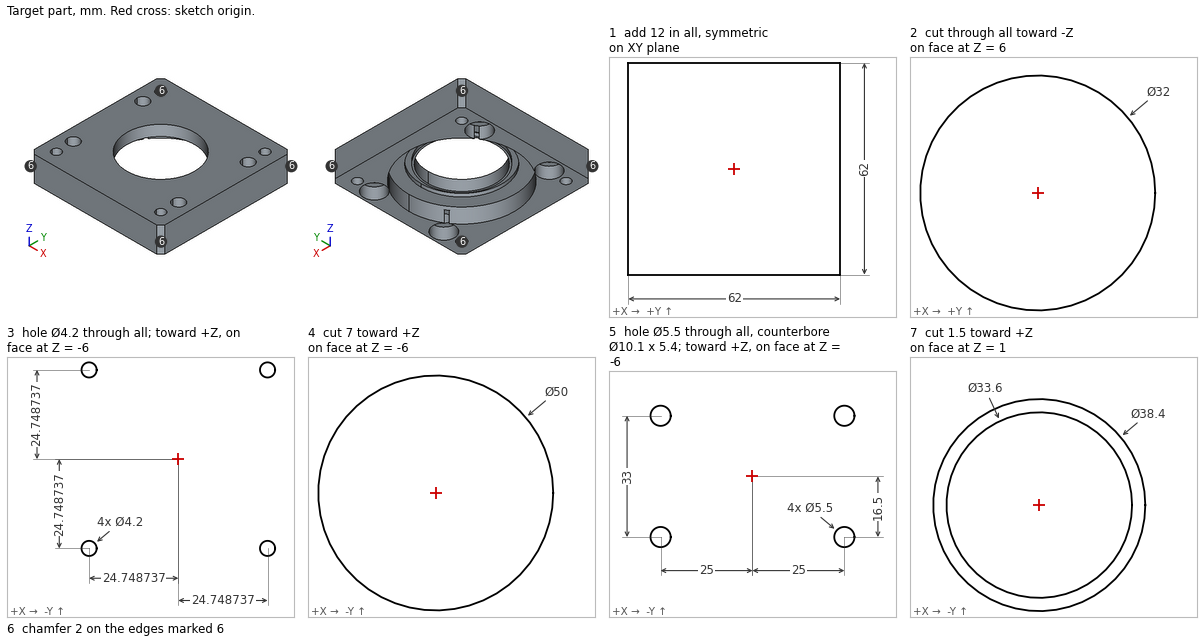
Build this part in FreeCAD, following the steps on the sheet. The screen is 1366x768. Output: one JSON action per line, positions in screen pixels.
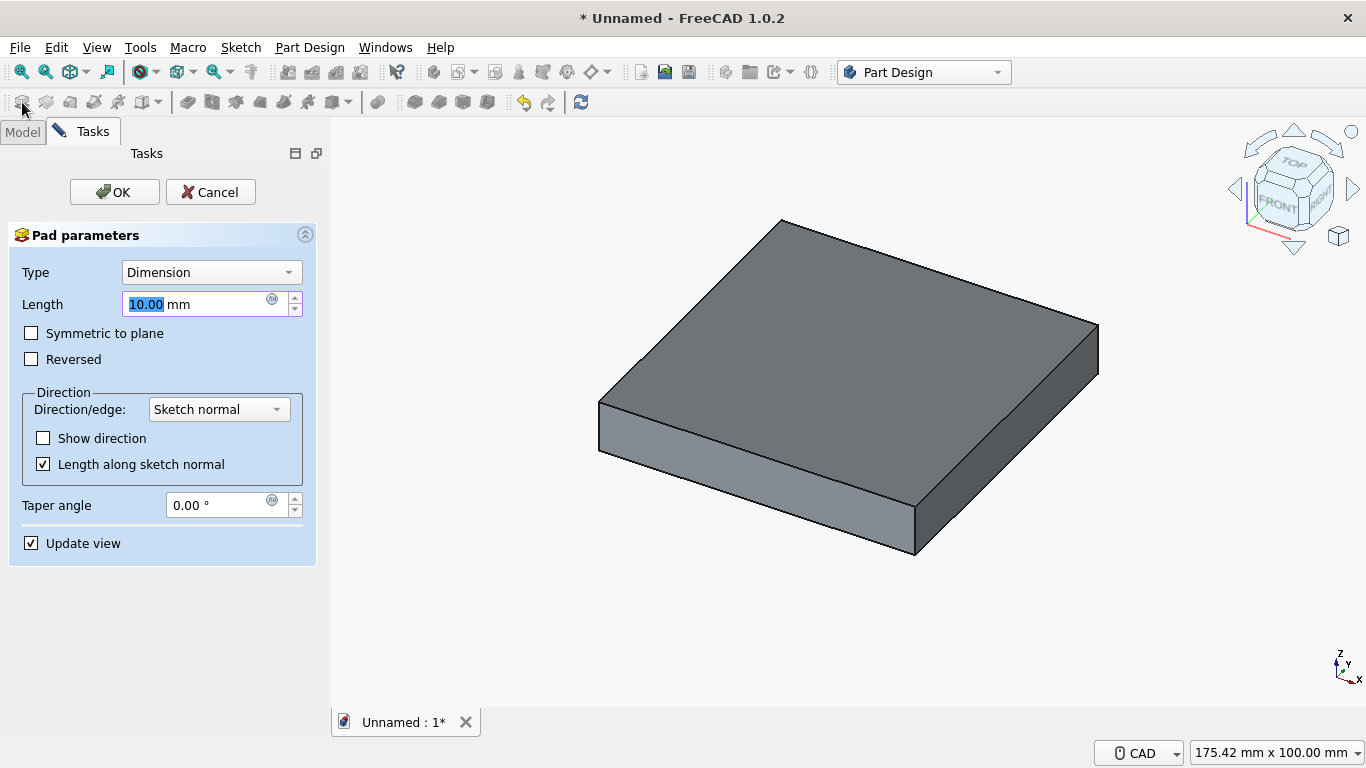
{"action": "type", "text": "12"}
{"action": "key", "text": "Tab"}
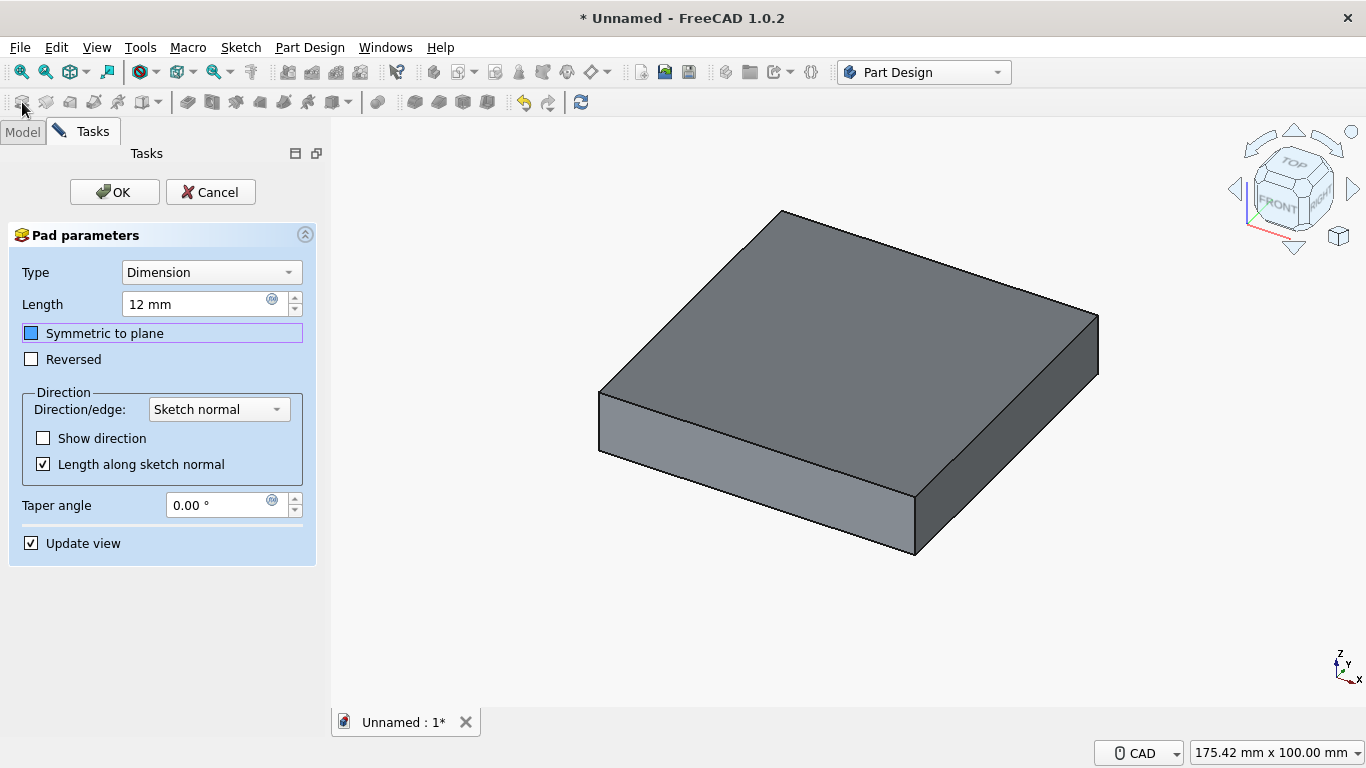
{"action": "left_click", "coordinate": [30, 333]}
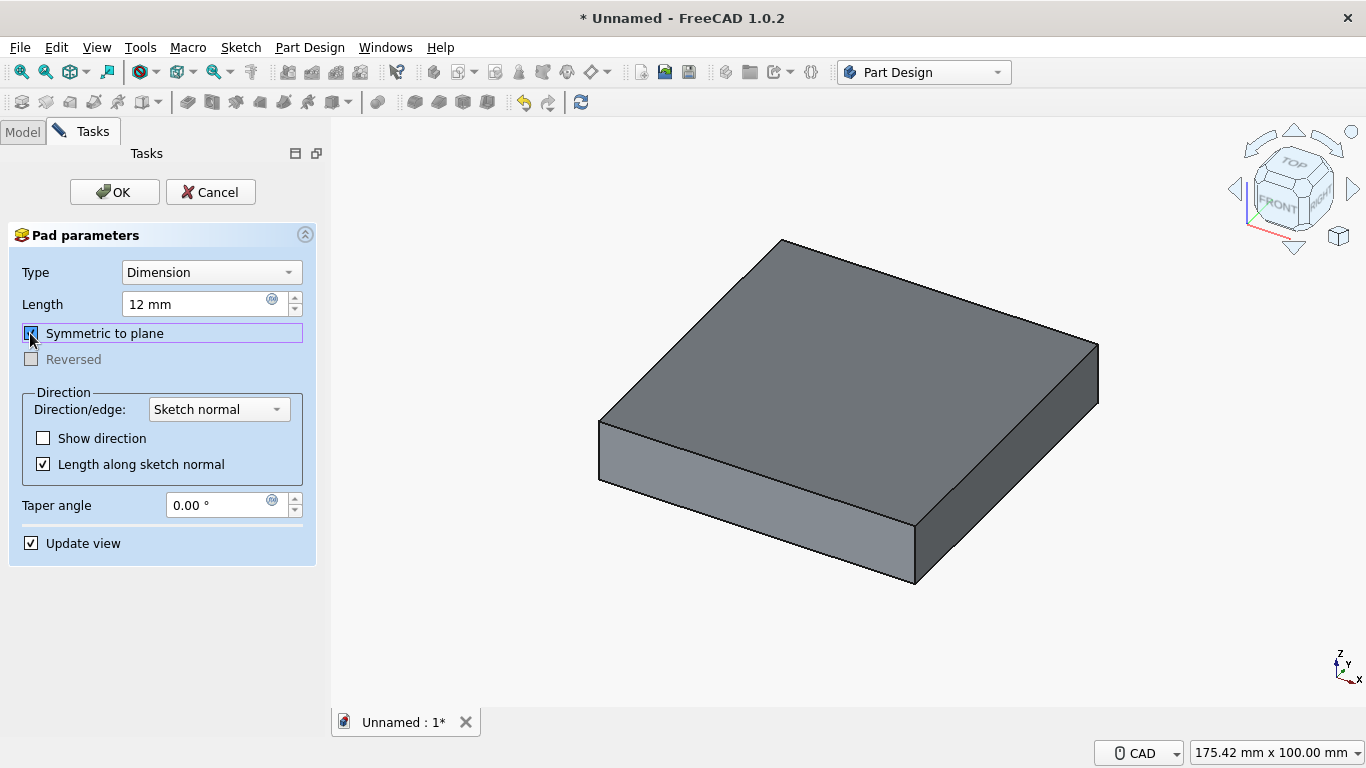
{"action": "left_click", "coordinate": [115, 192]}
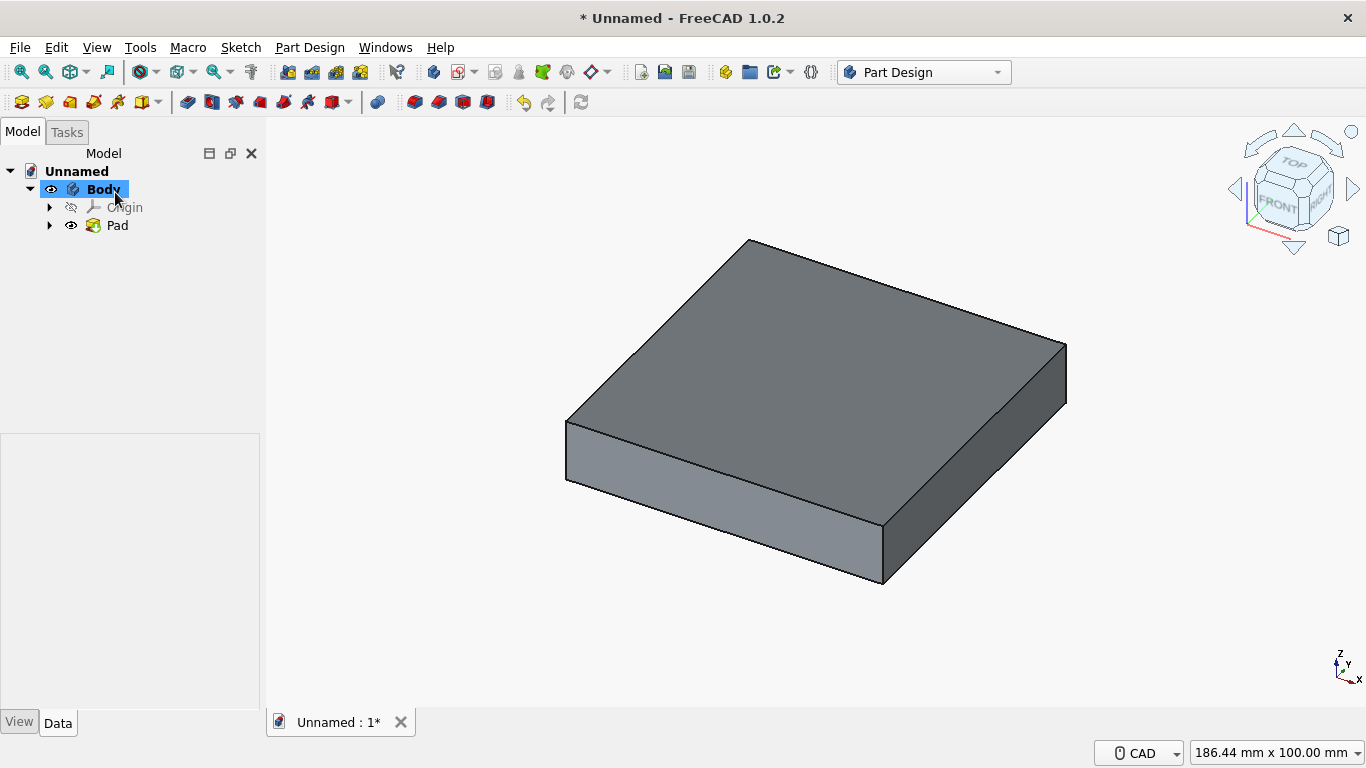
{"action": "left_click", "coordinate": [816, 382]}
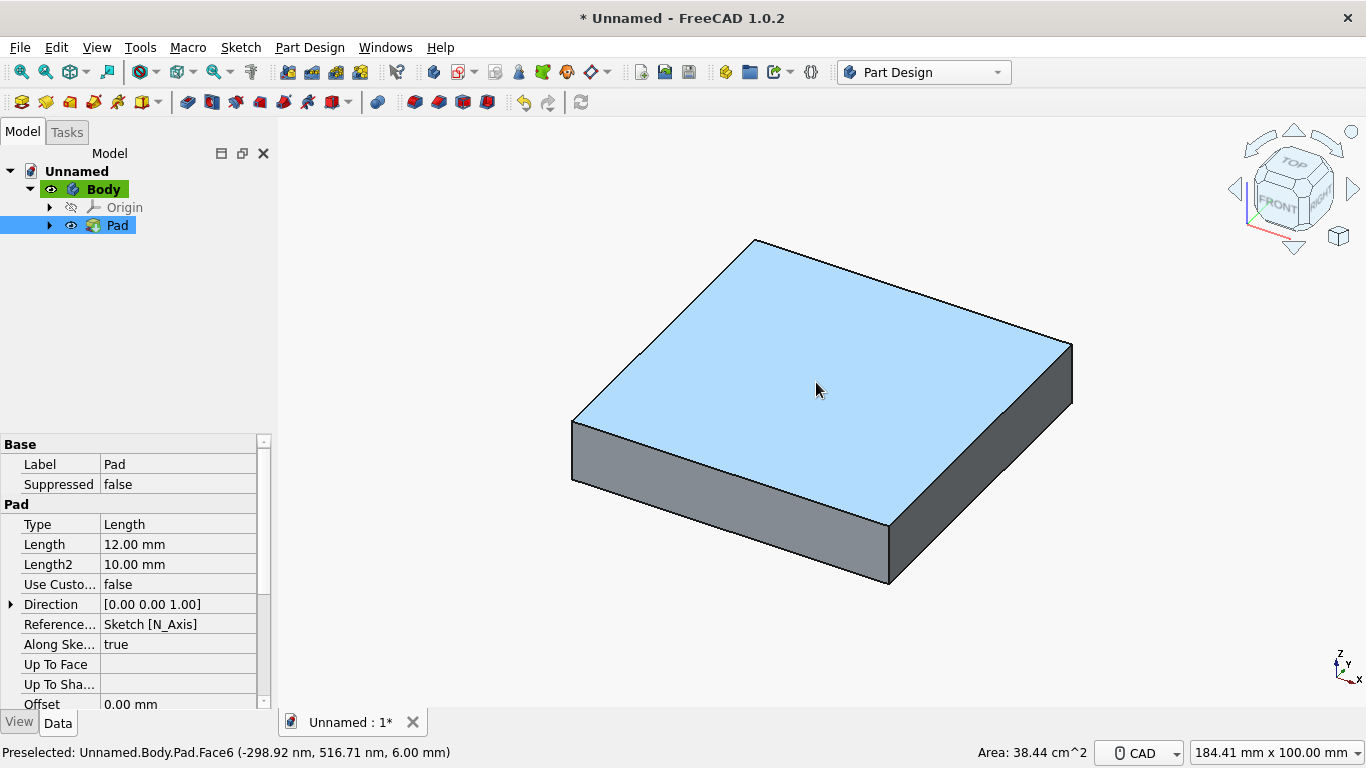
{"action": "left_click", "coordinate": [458, 72]}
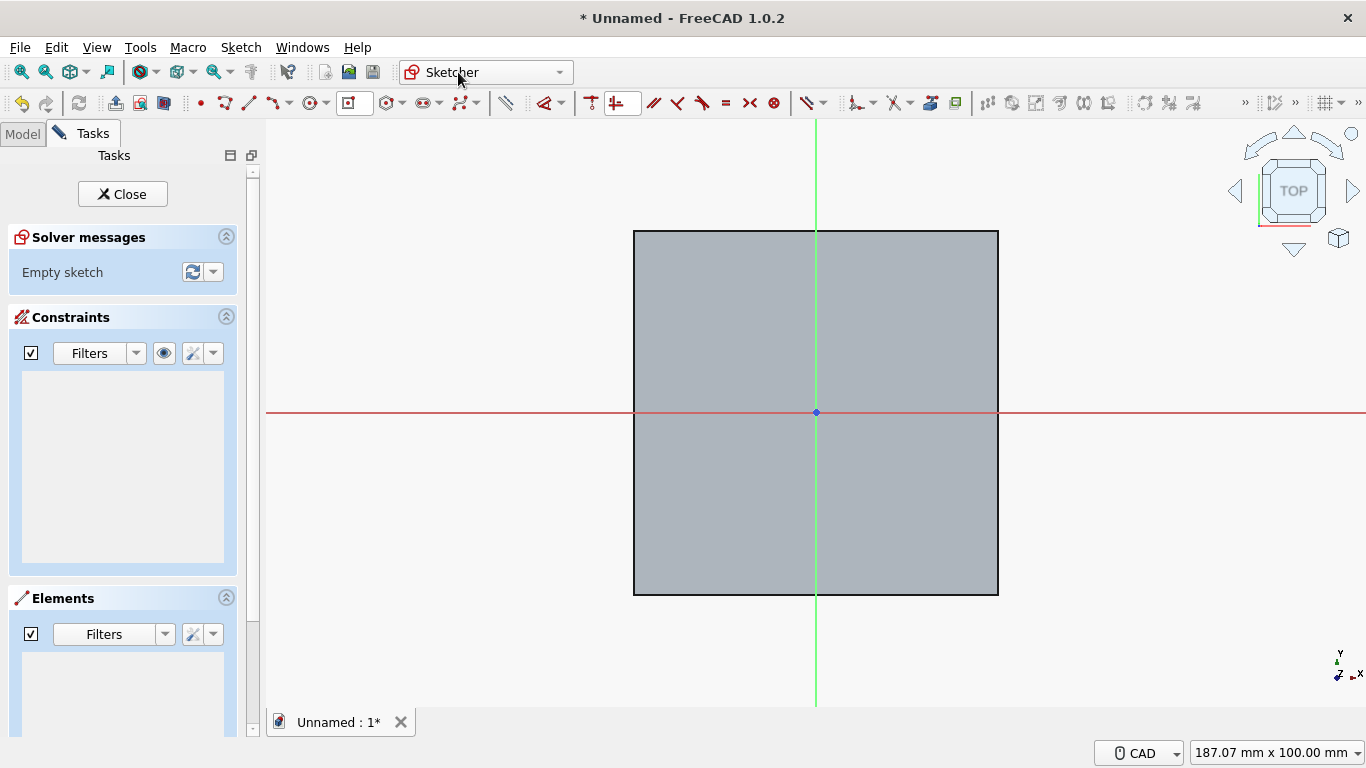
{"action": "scroll", "coordinate": [899, 413], "scroll_direction": "up", "scroll_amount": 3}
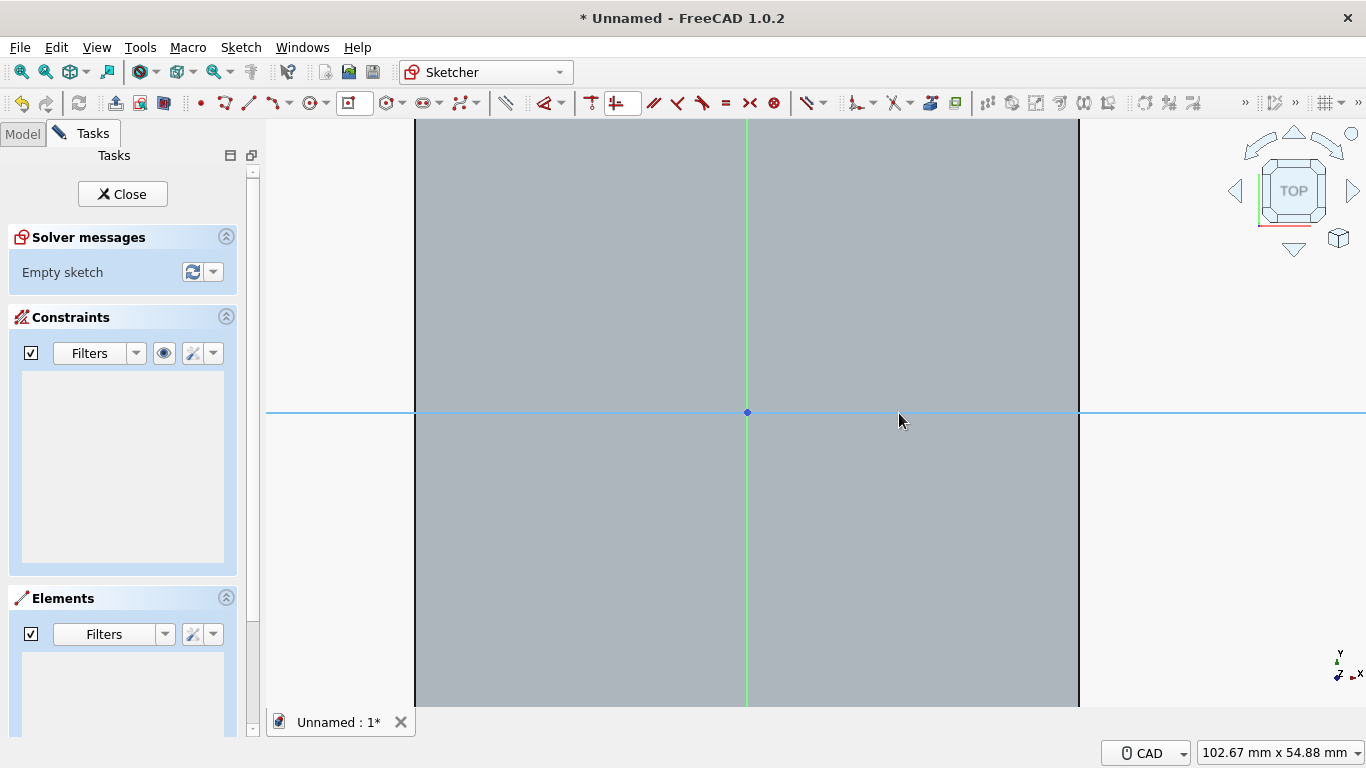
{"action": "left_click", "coordinate": [310, 104]}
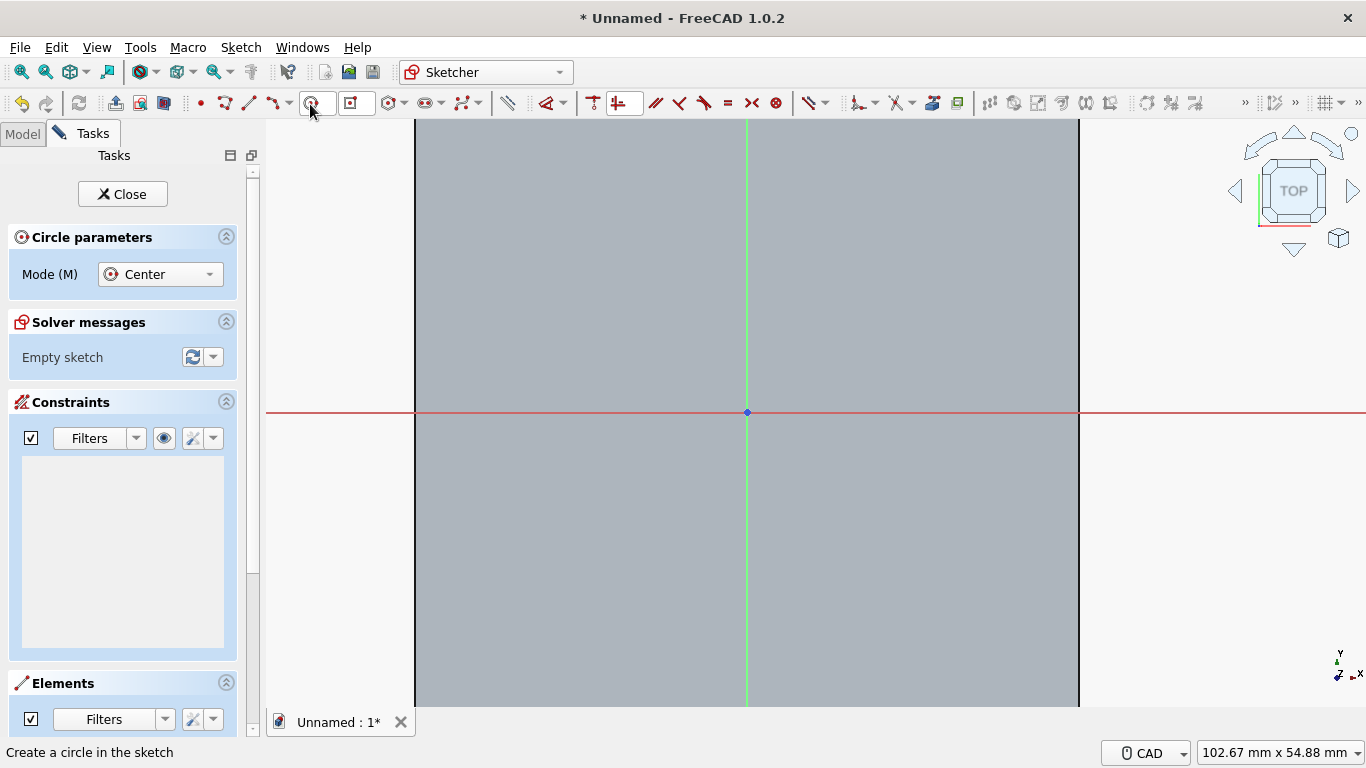
{"action": "left_click", "coordinate": [747, 413]}
{"action": "mouse_move", "coordinate": [869, 291]}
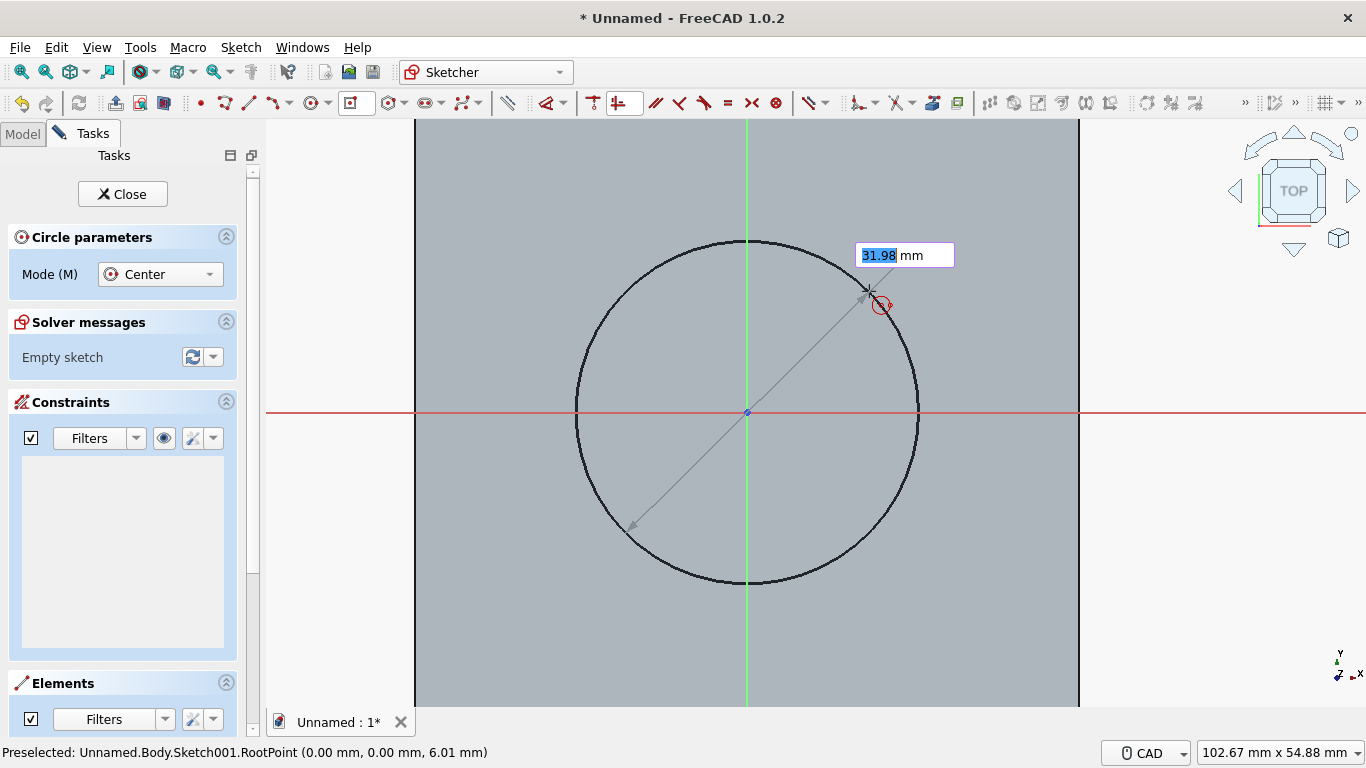
{"action": "type", "text": "32"}
{"action": "key", "text": "Return"}
{"action": "key", "text": "Escape"}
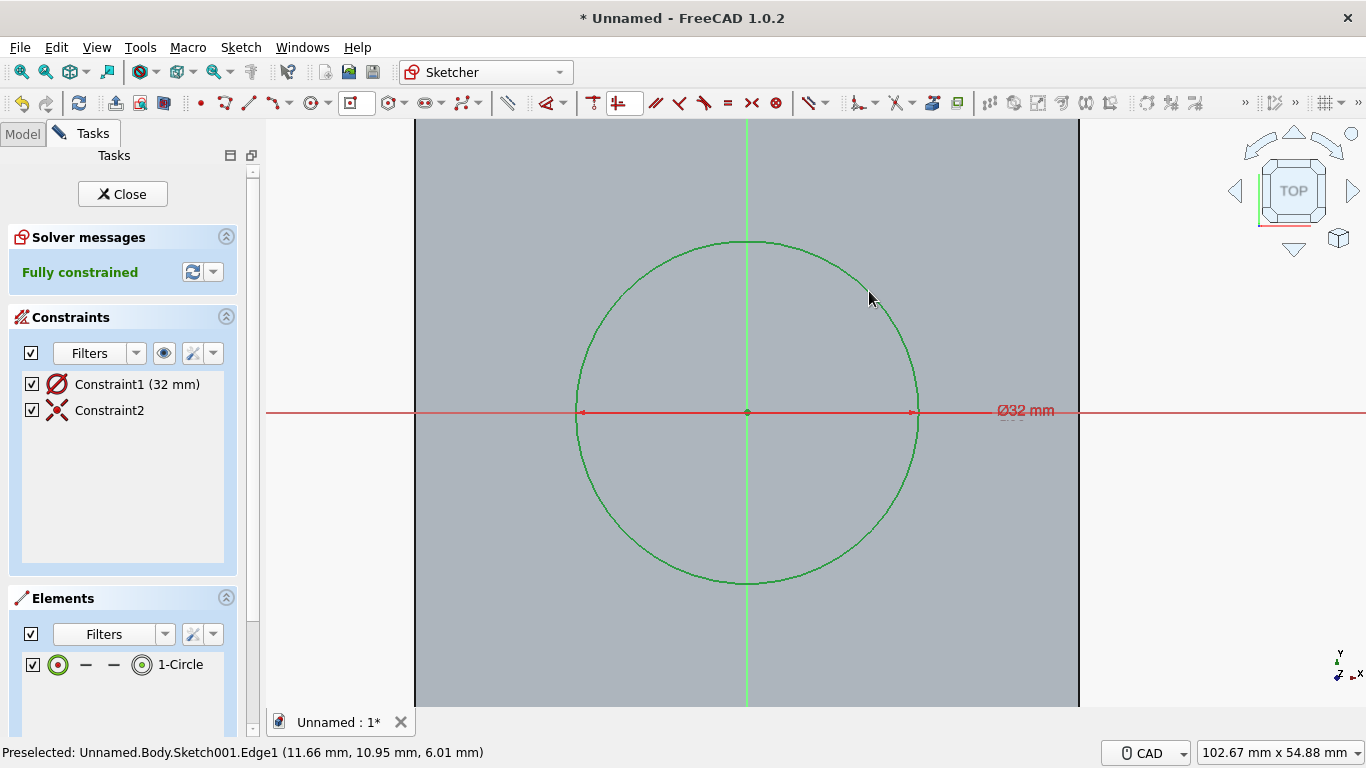
{"action": "left_click", "coordinate": [123, 194]}